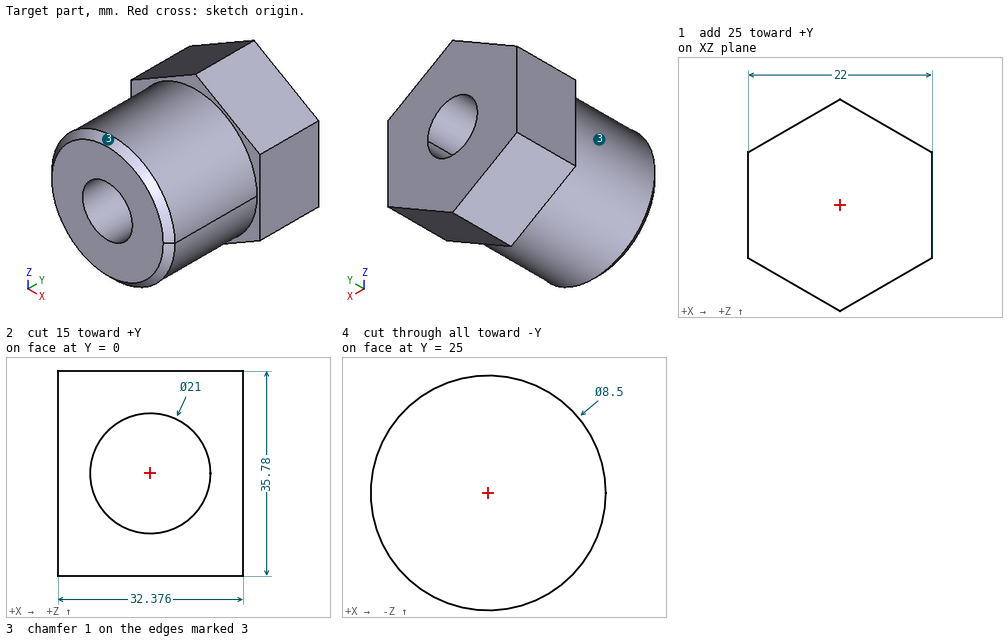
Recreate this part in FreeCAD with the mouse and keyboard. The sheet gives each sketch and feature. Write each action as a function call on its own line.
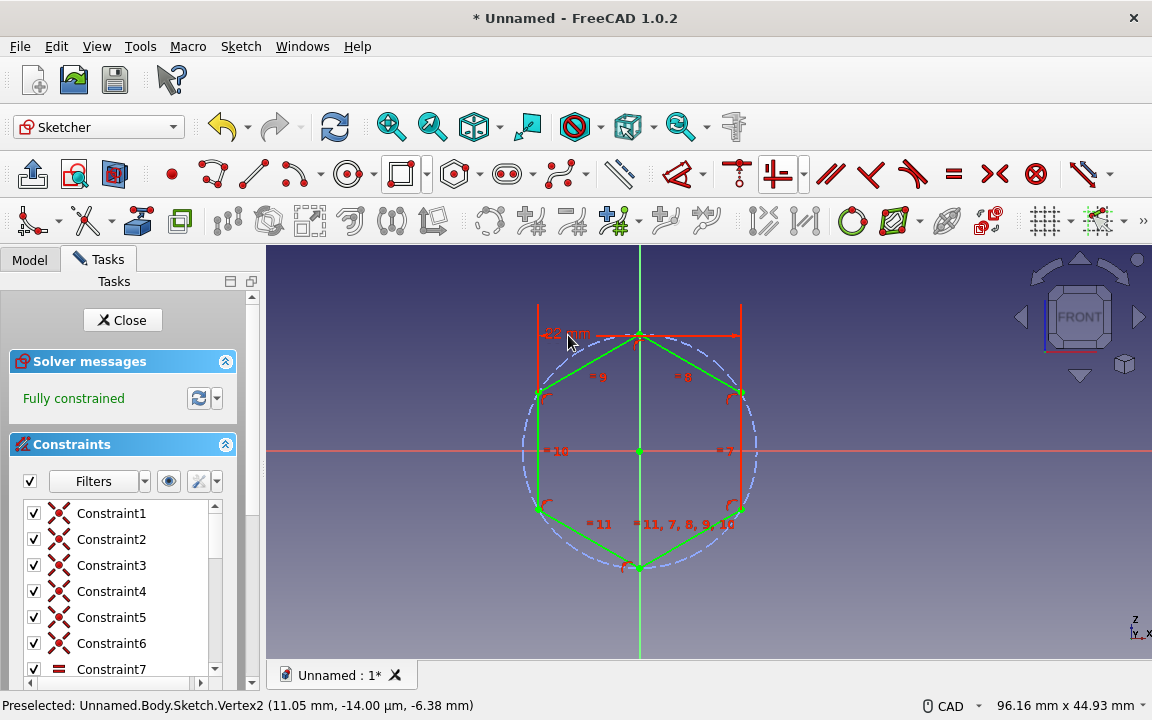
click(123, 320)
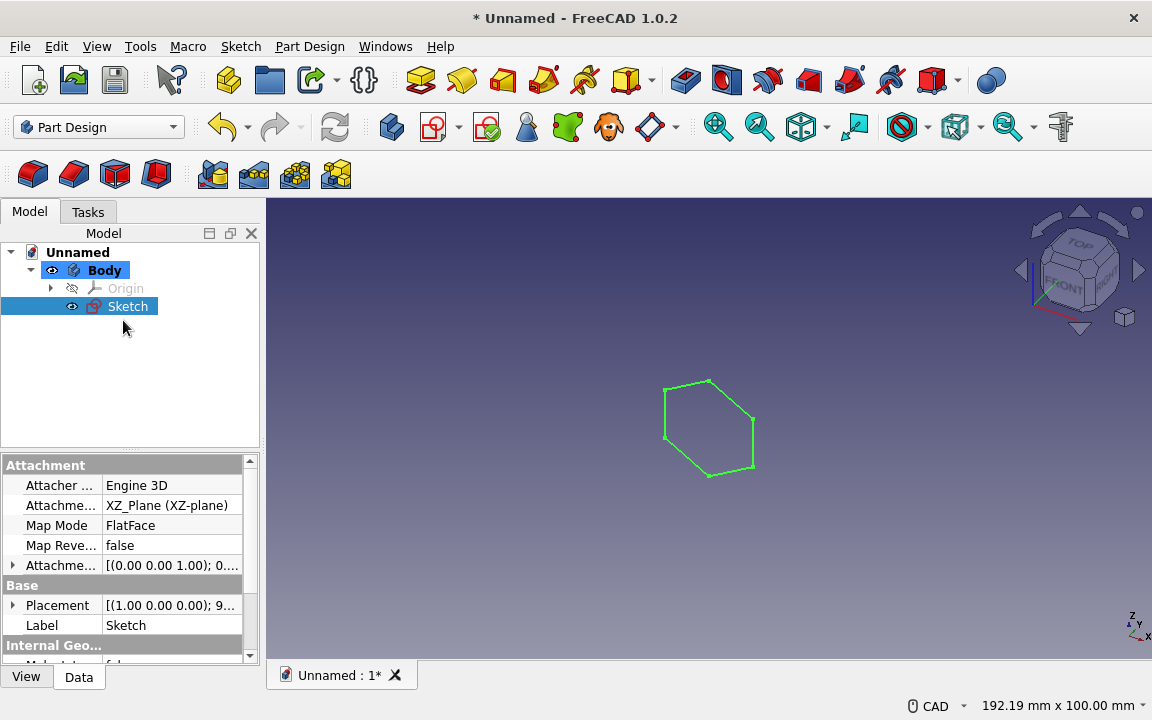
click(421, 80)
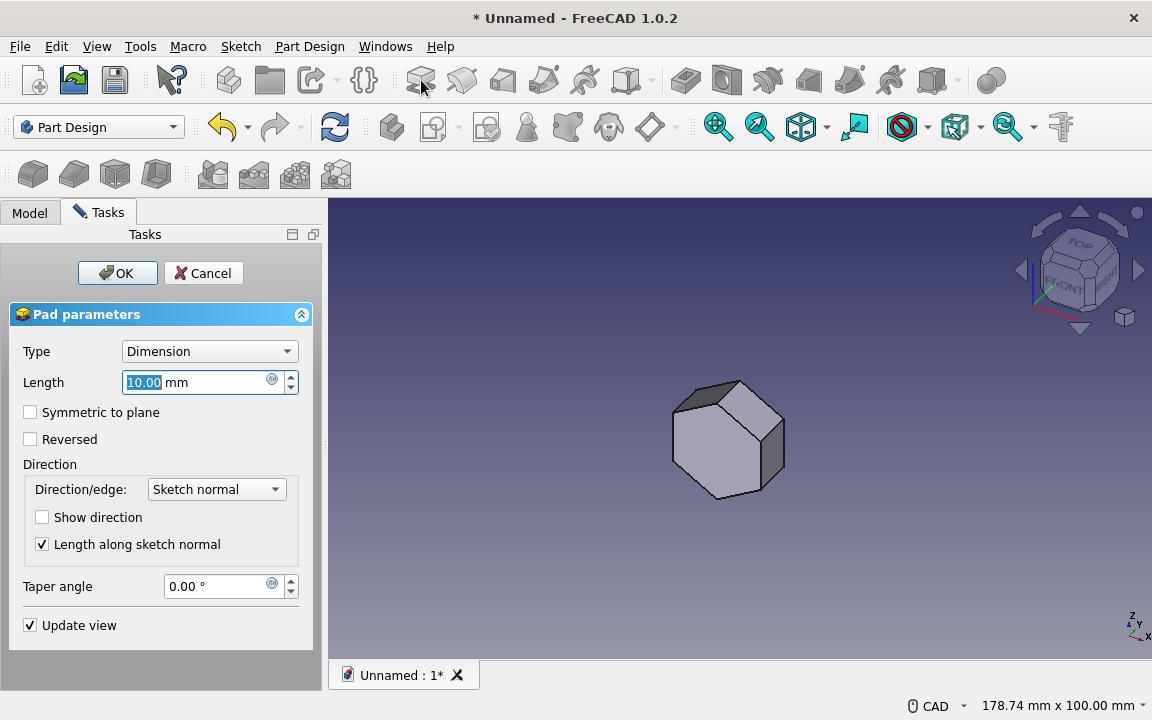
text(25)
key(Tab)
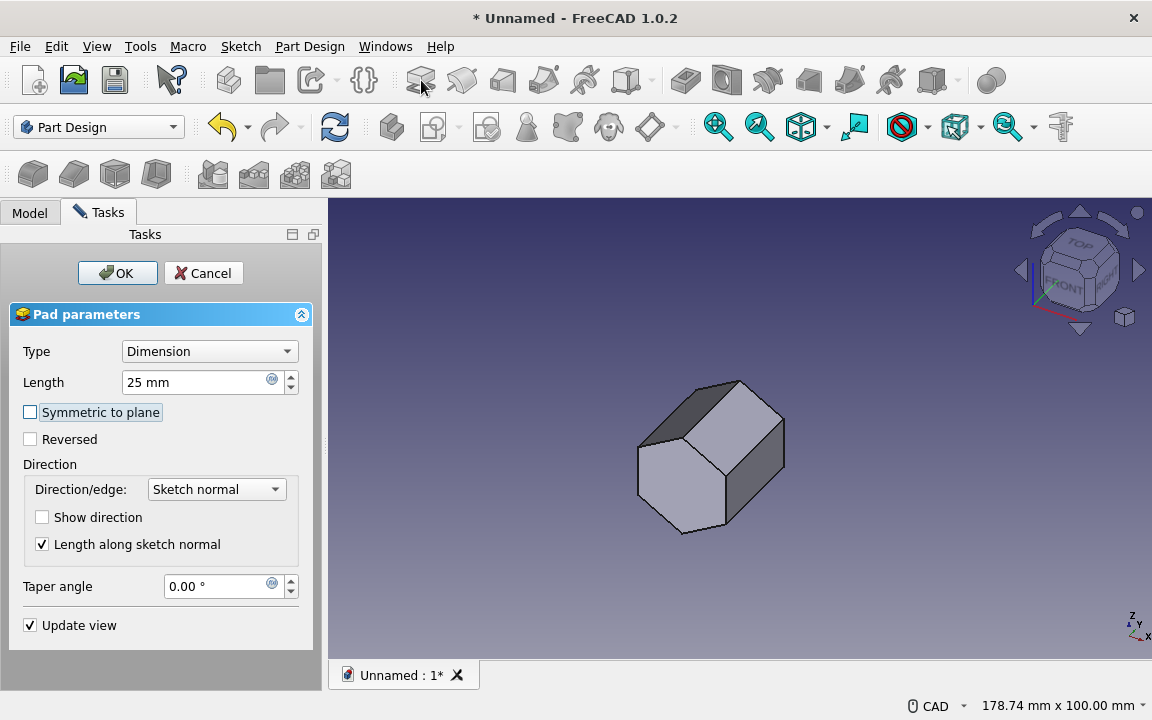
click(31, 439)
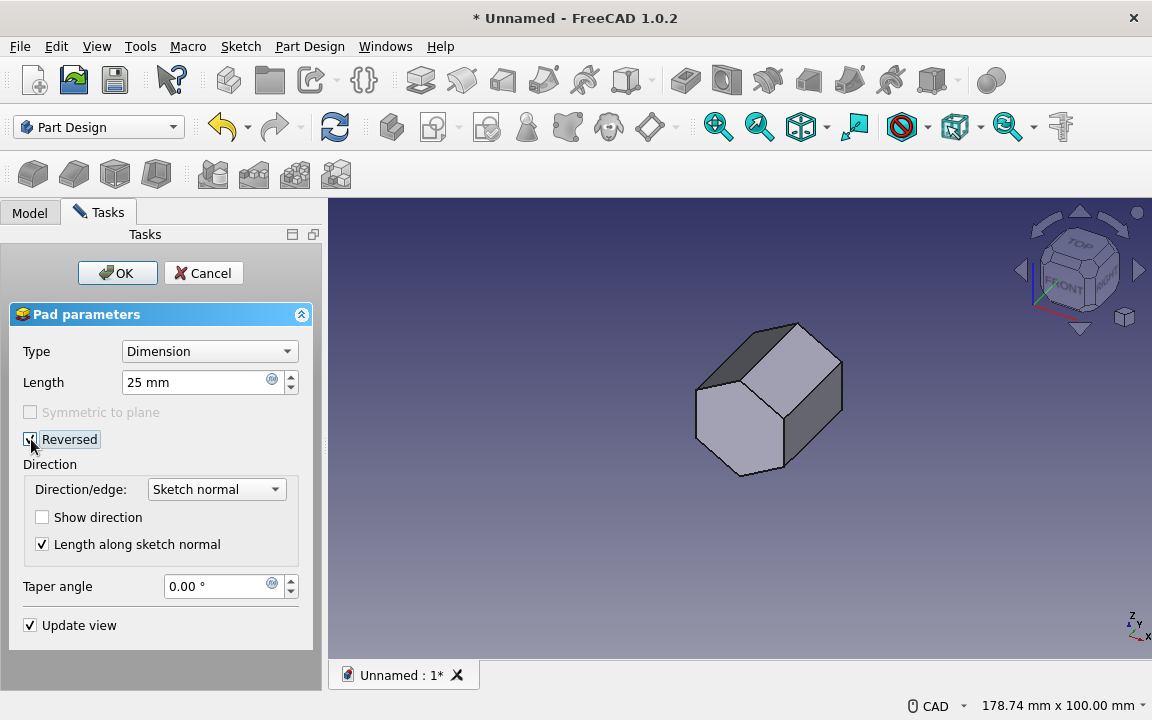
click(118, 273)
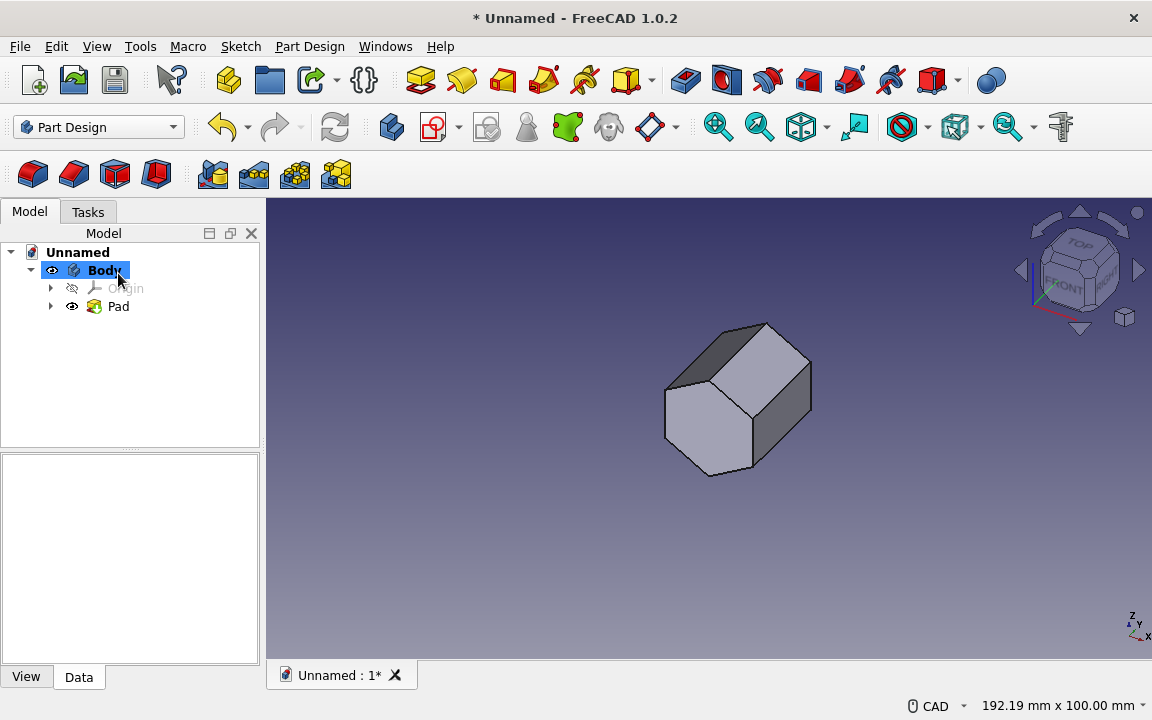
click(719, 128)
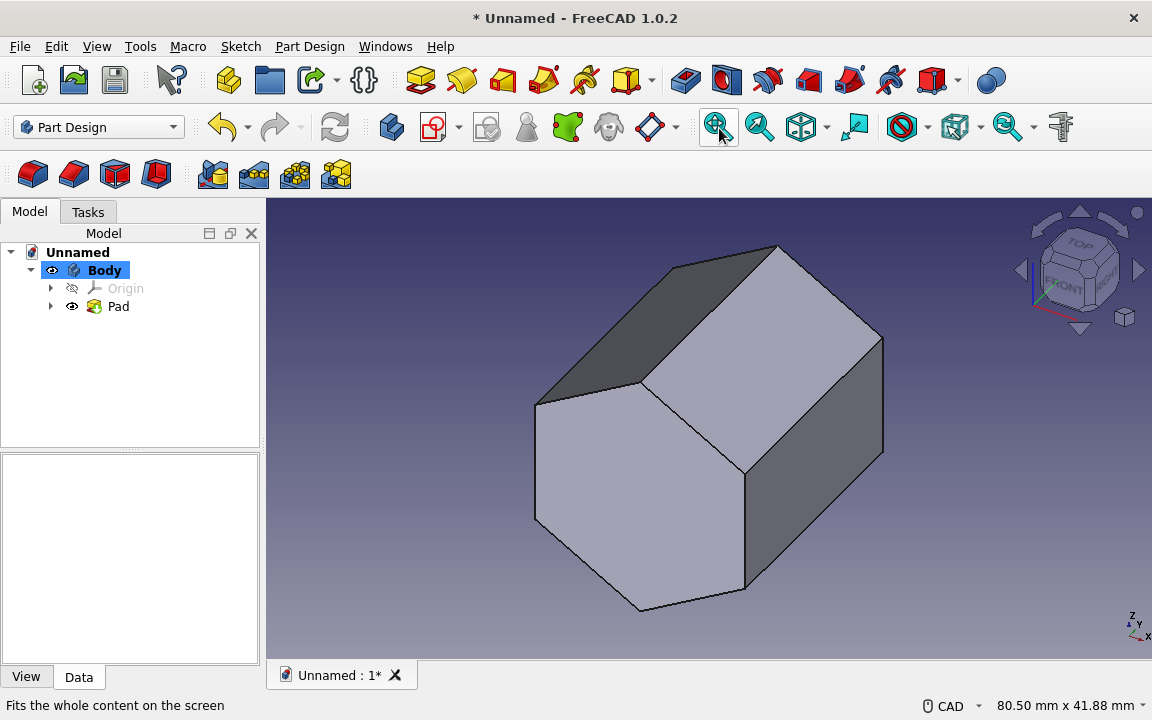
click(640, 496)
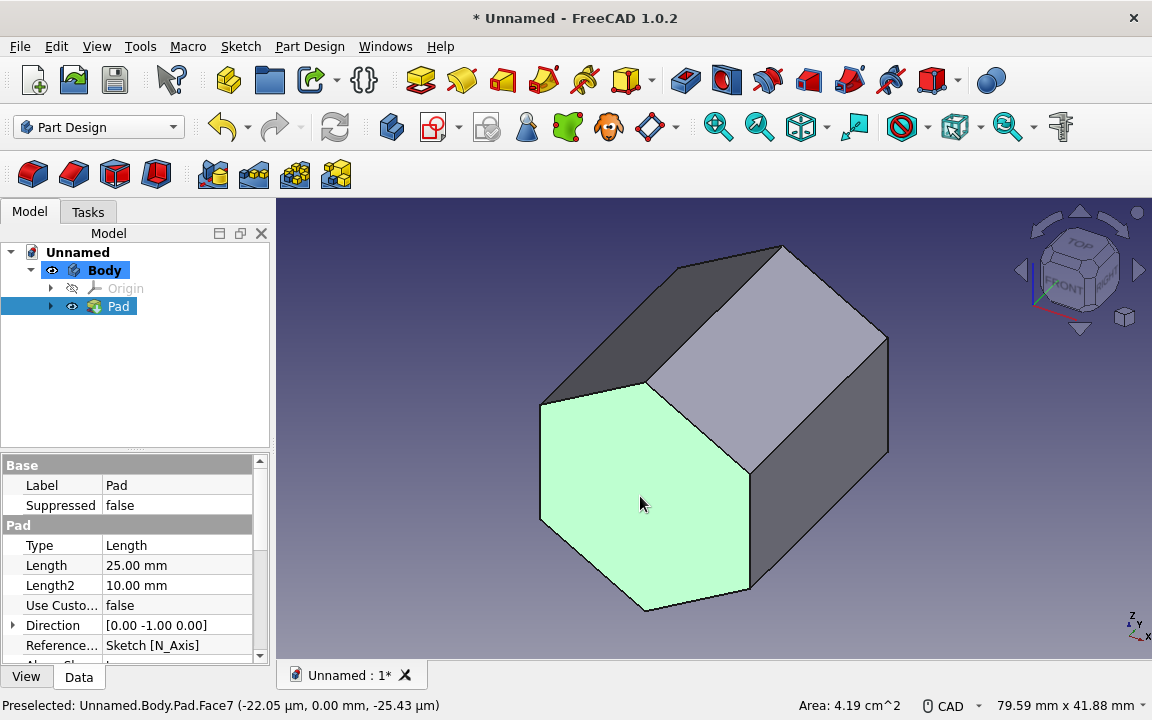
click(432, 128)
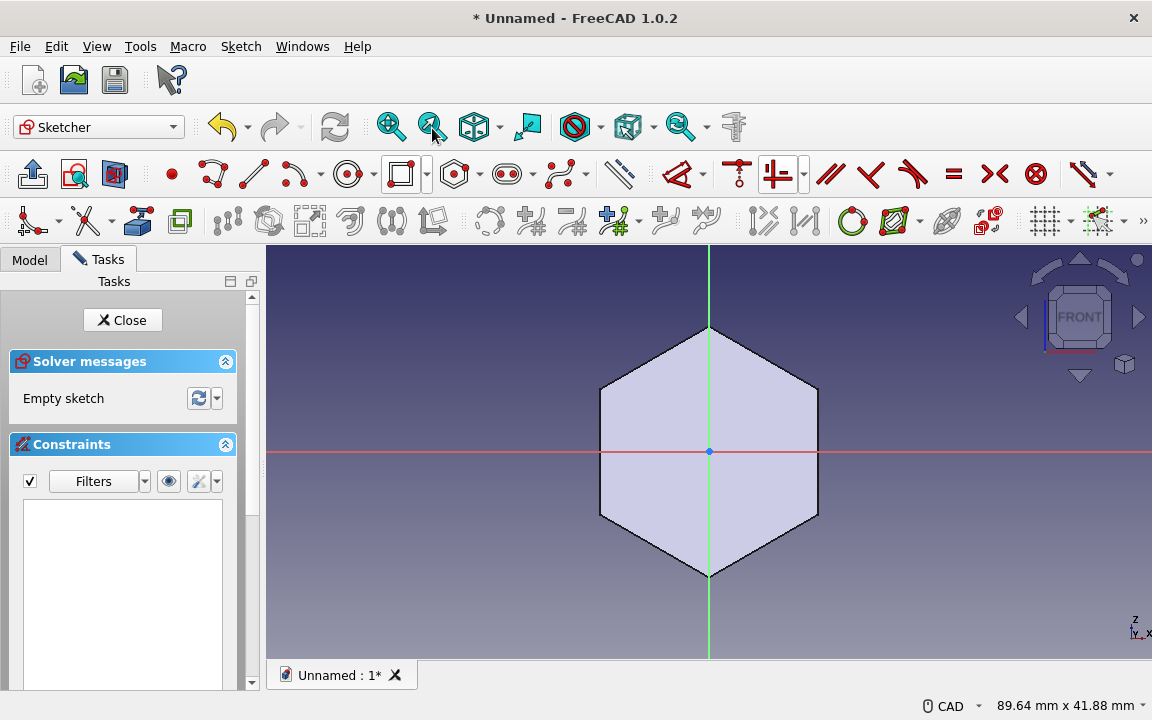
scroll(501, 452, down, 2)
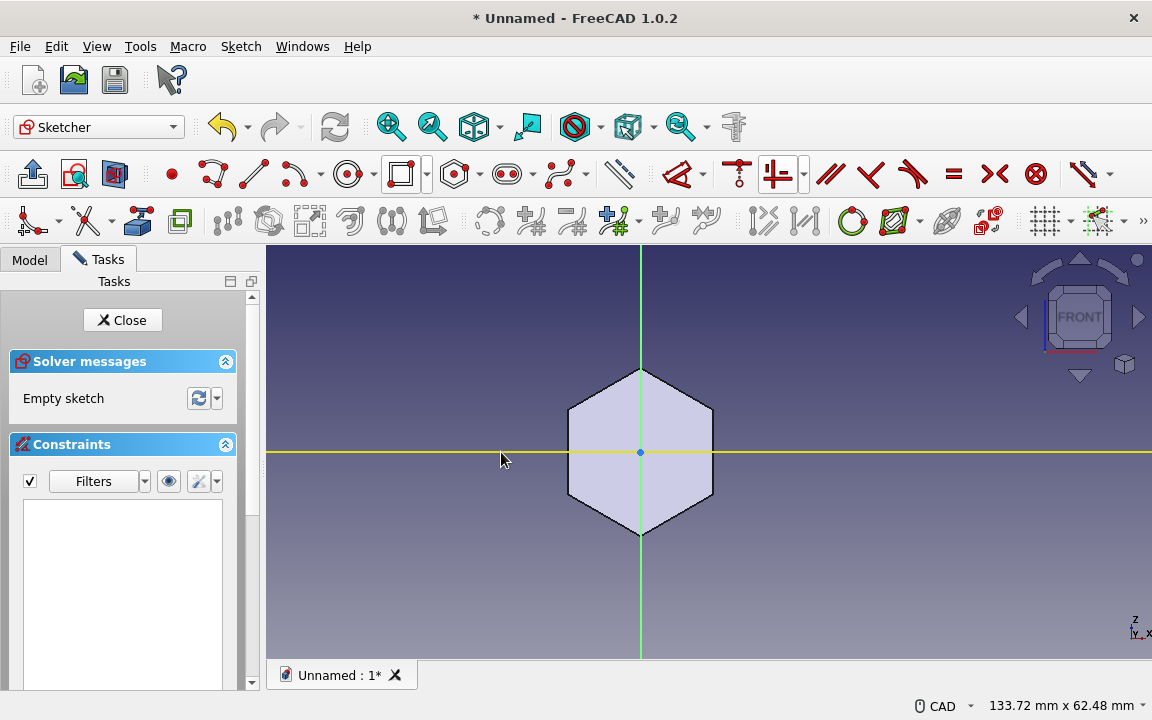
key(g)
key(v)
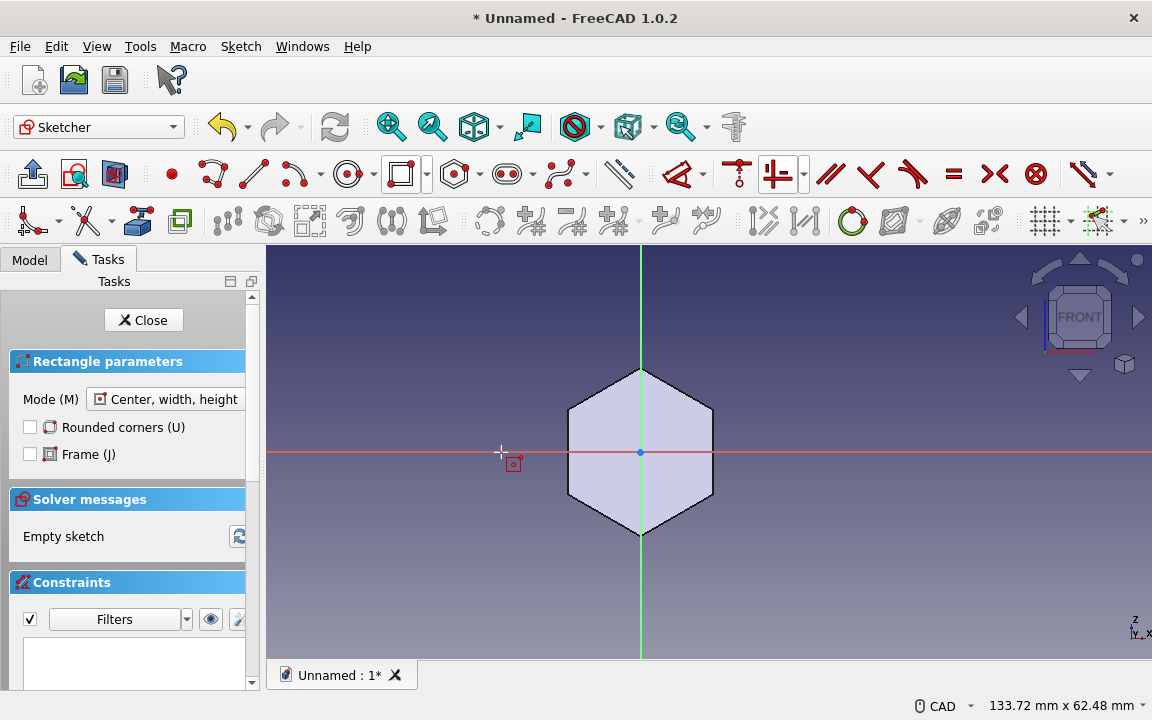
click(641, 452)
move(748, 334)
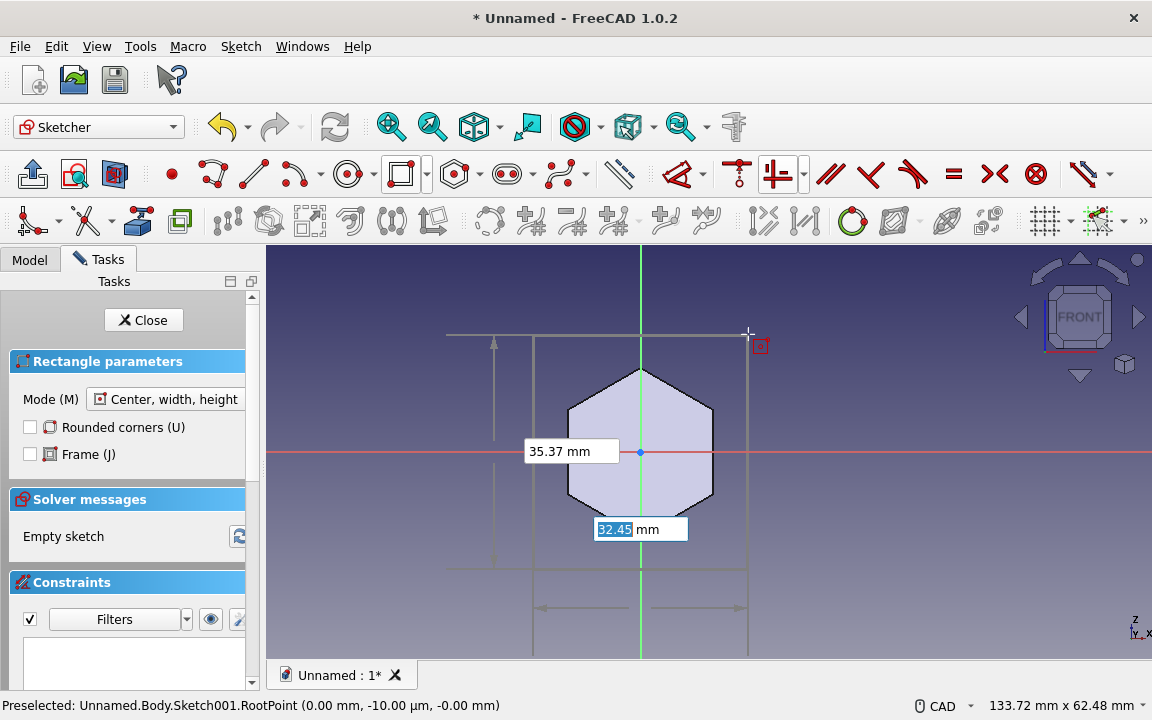
text(32.376)
key(Tab)
text(35.78)
key(Return)